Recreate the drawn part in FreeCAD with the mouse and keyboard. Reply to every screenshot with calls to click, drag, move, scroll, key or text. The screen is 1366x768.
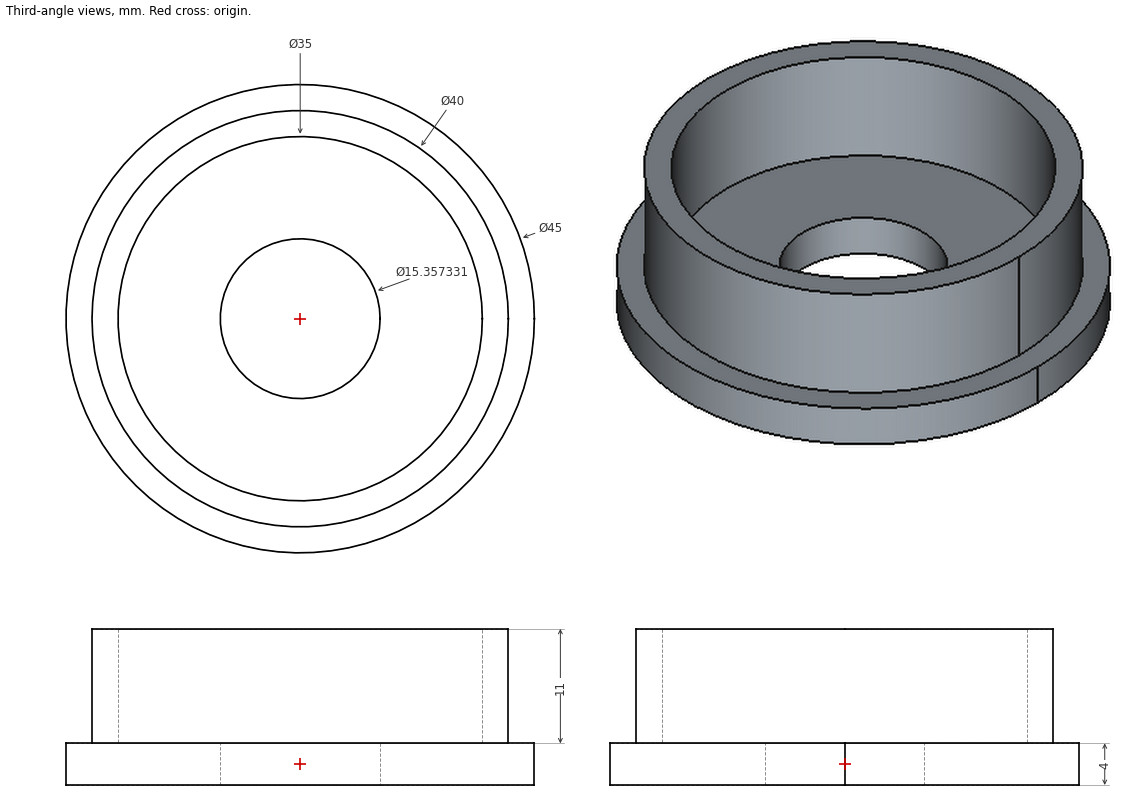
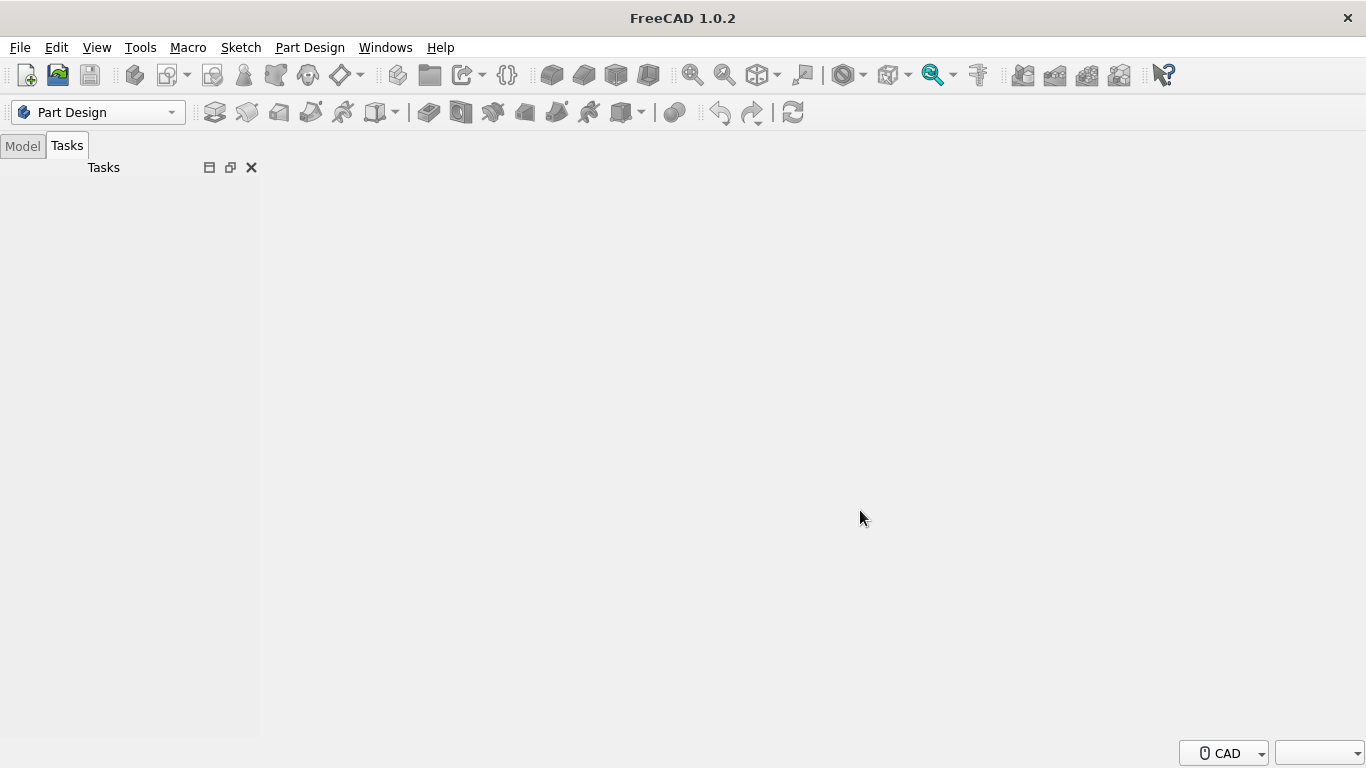
key(ctrl+n)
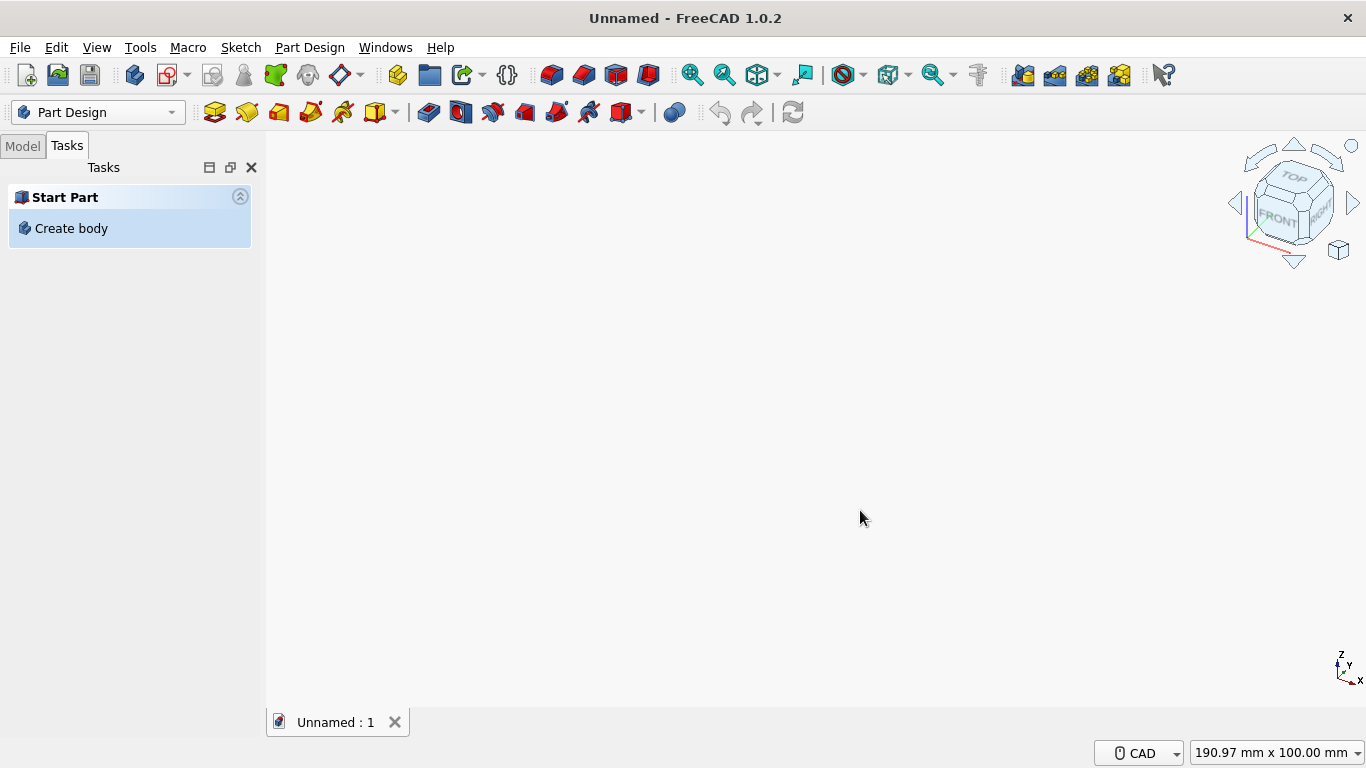
click(168, 76)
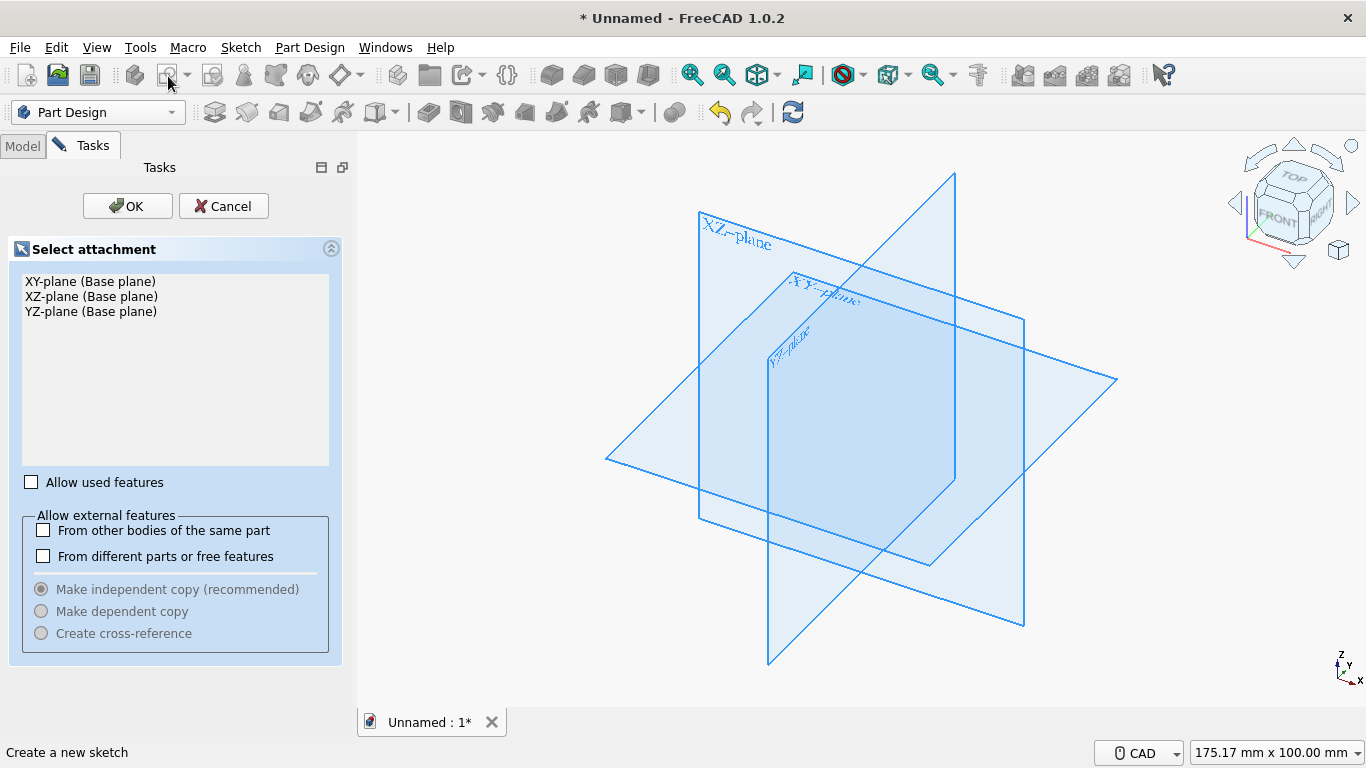
click(82, 282)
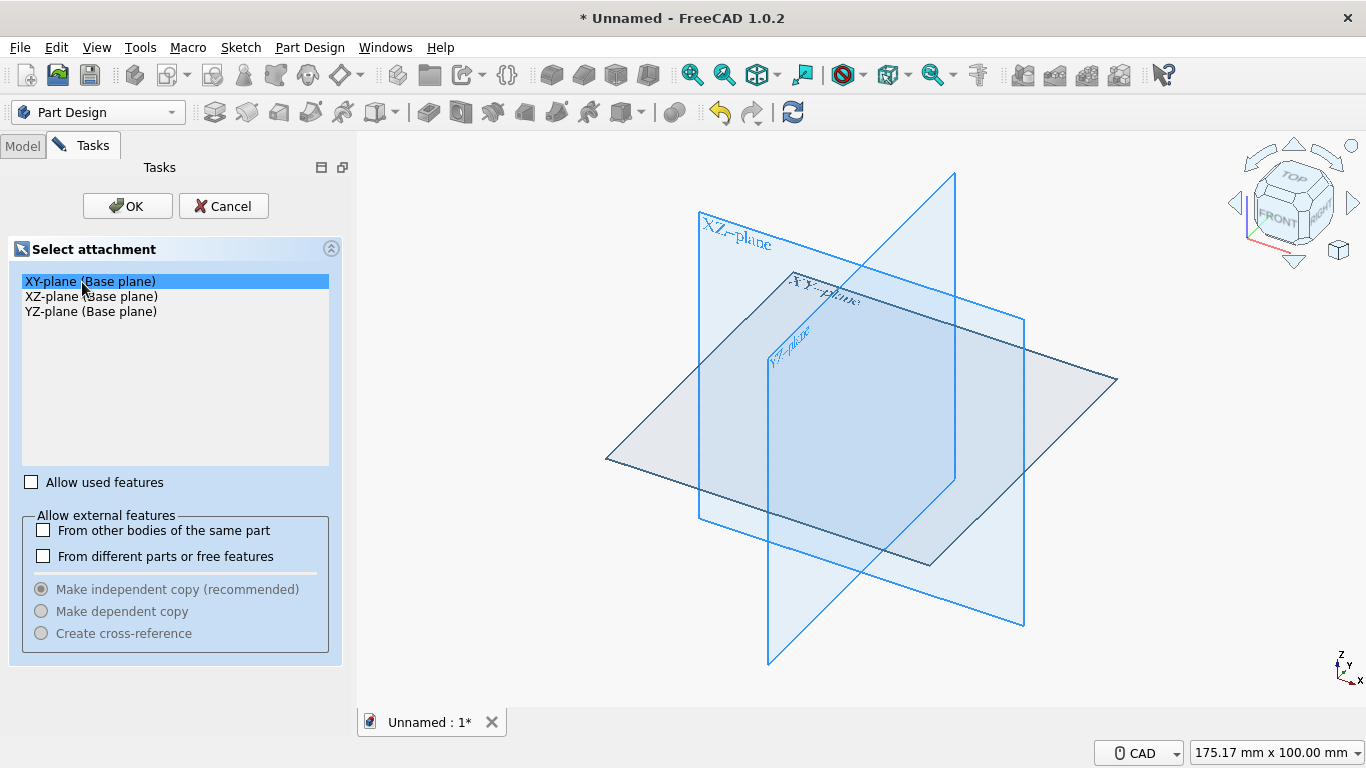
click(128, 206)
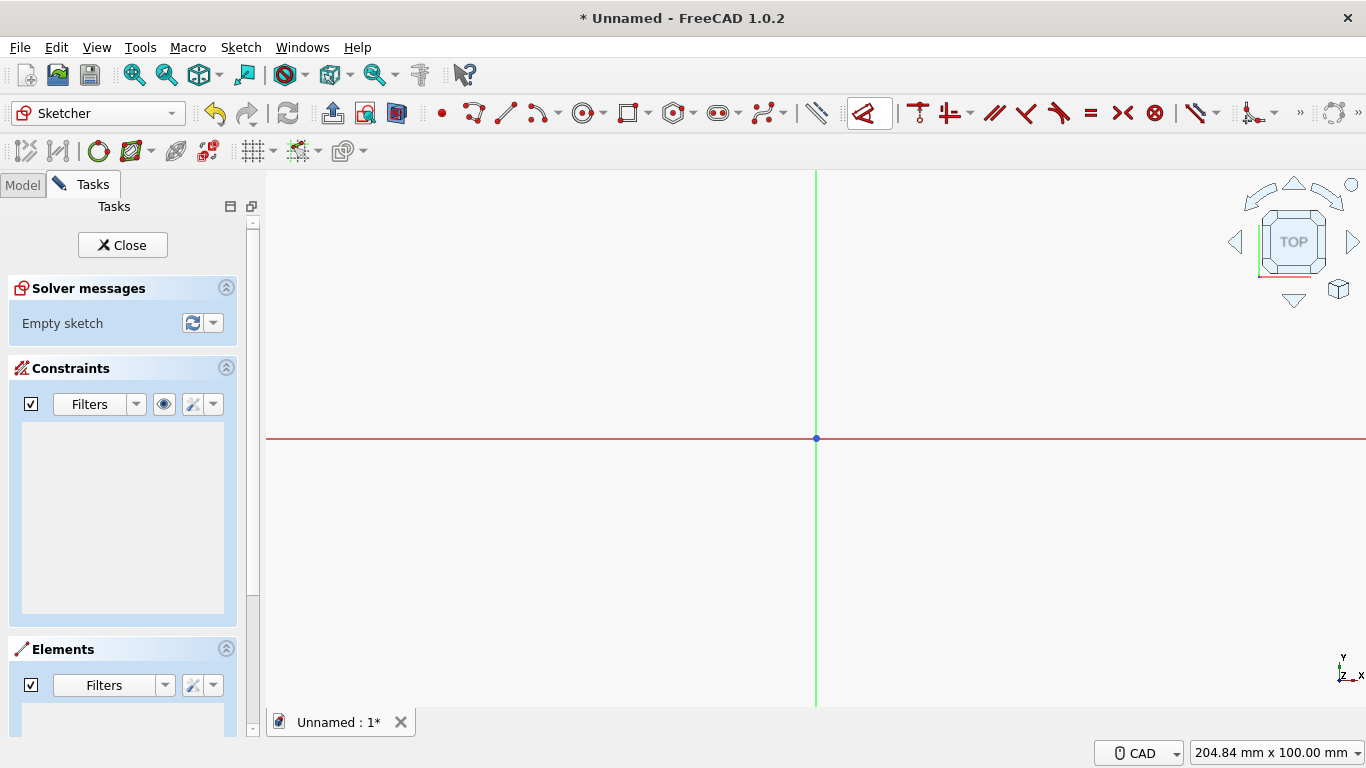
scroll(955, 439, up, 2)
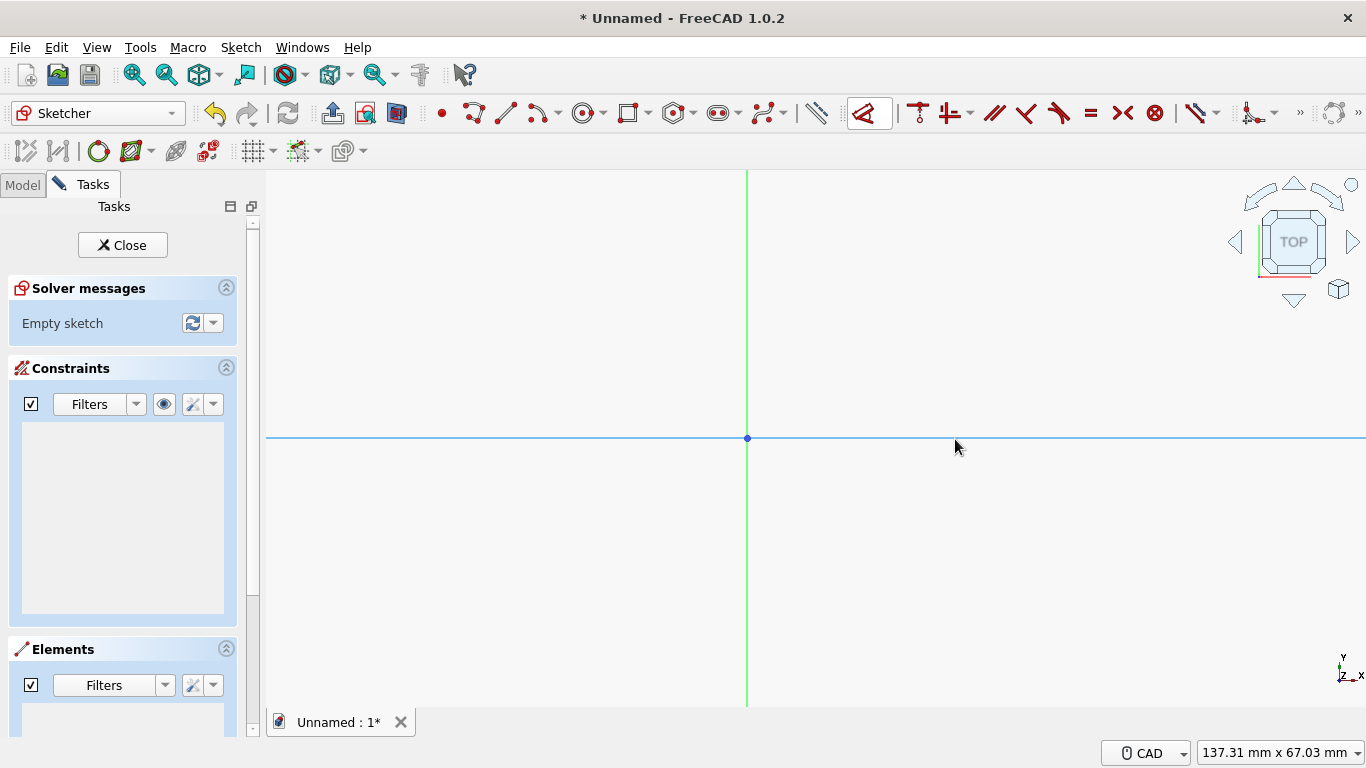
click(584, 114)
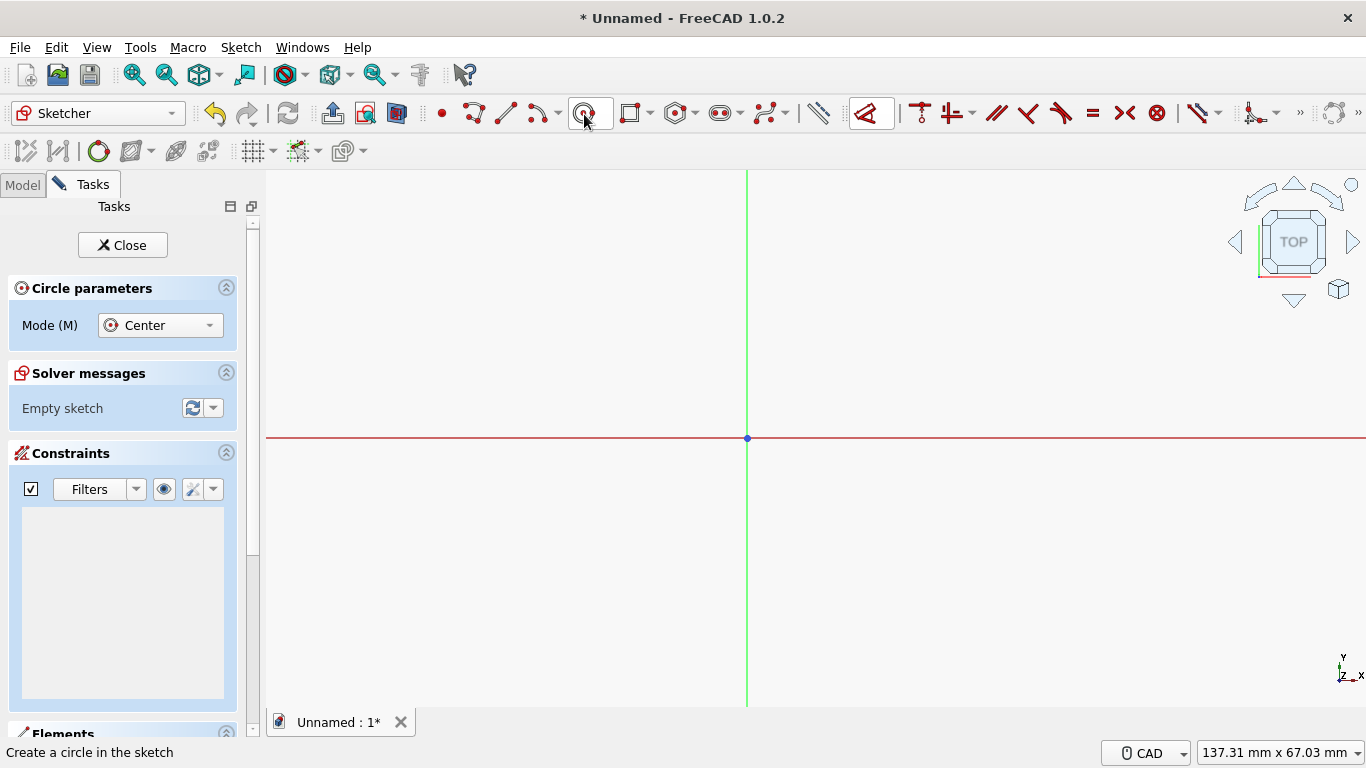
click(747, 438)
click(875, 311)
key(Escape)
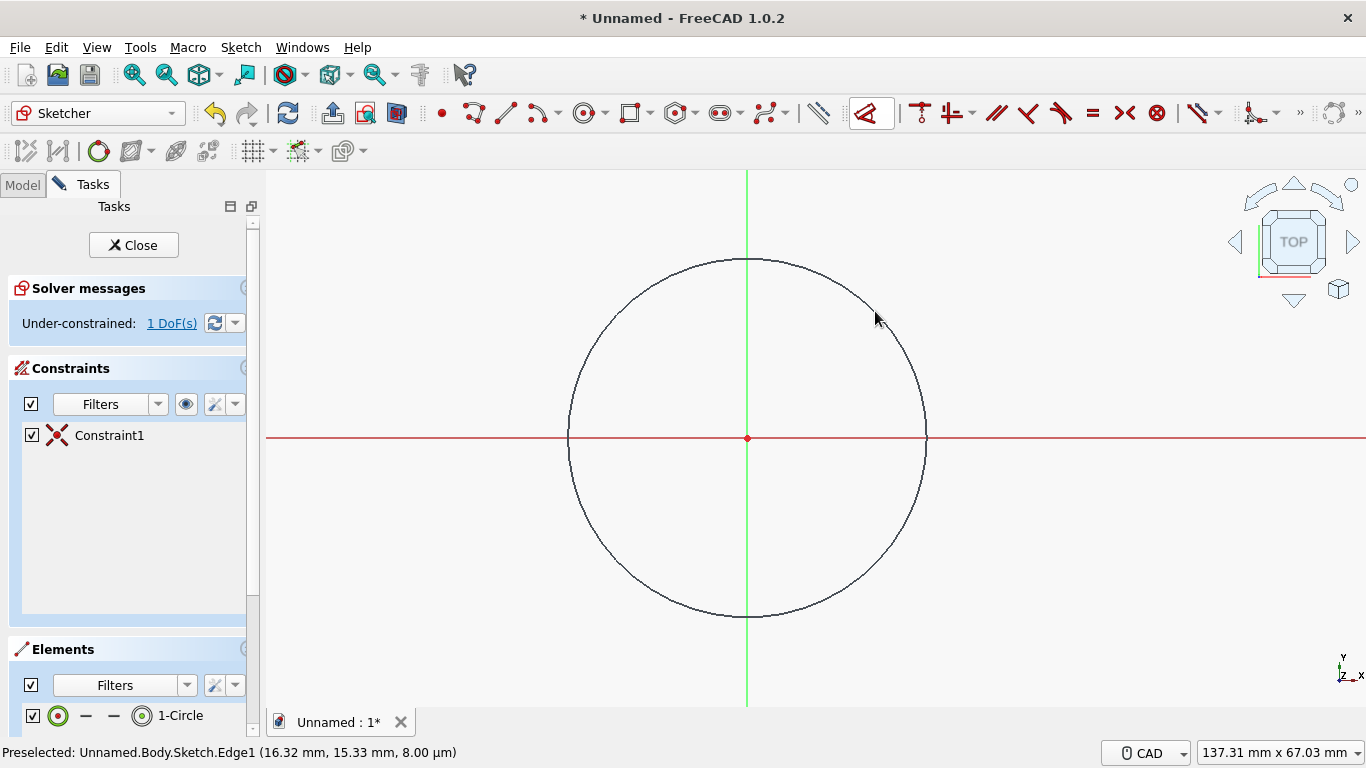
key(d)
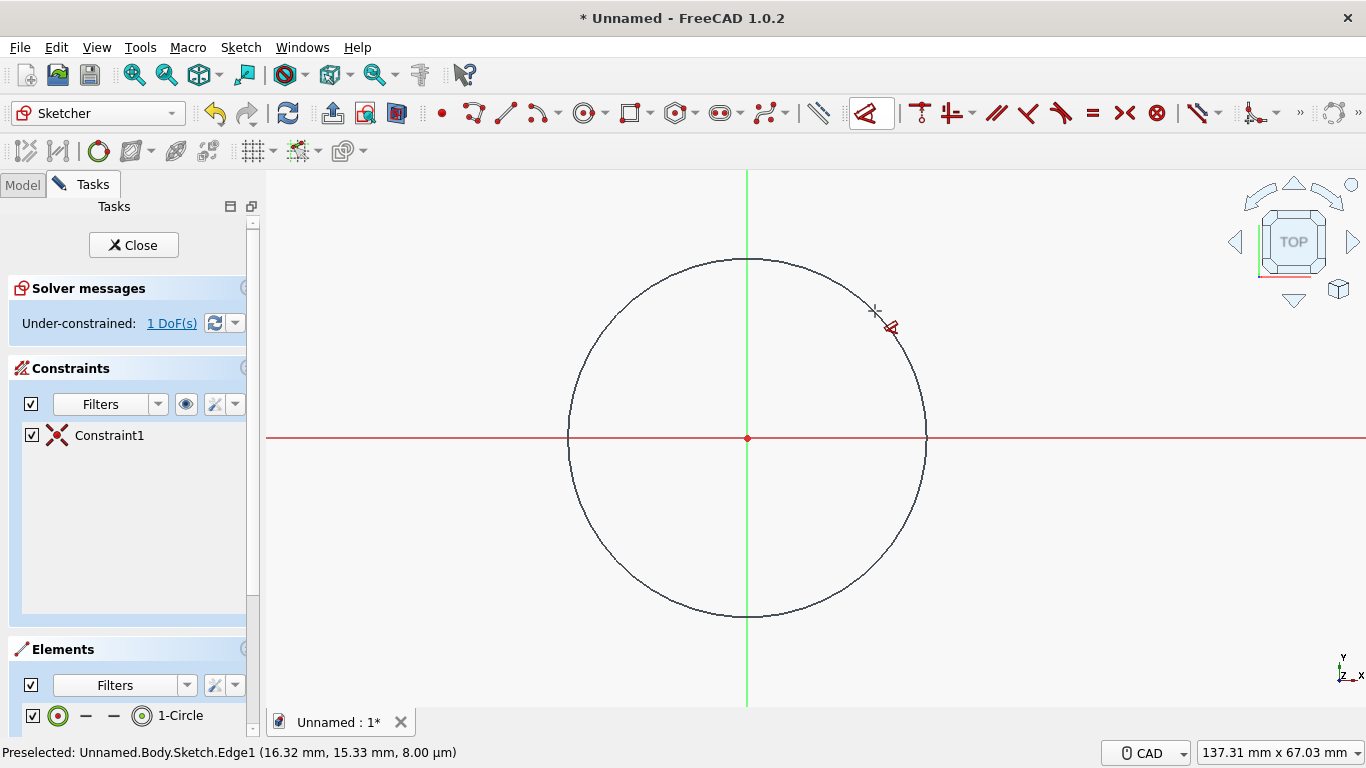
click(874, 311)
click(897, 288)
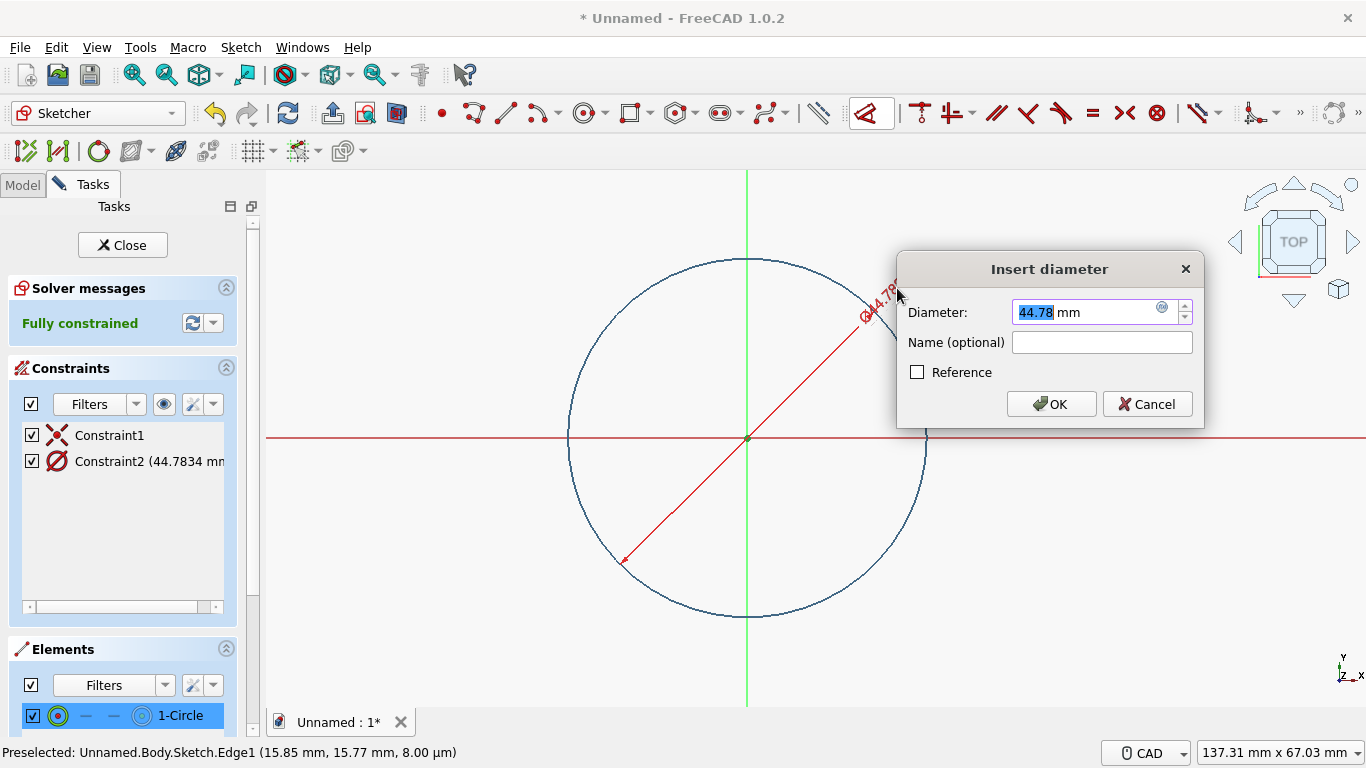
text(45)
key(Return)
key(Escape)